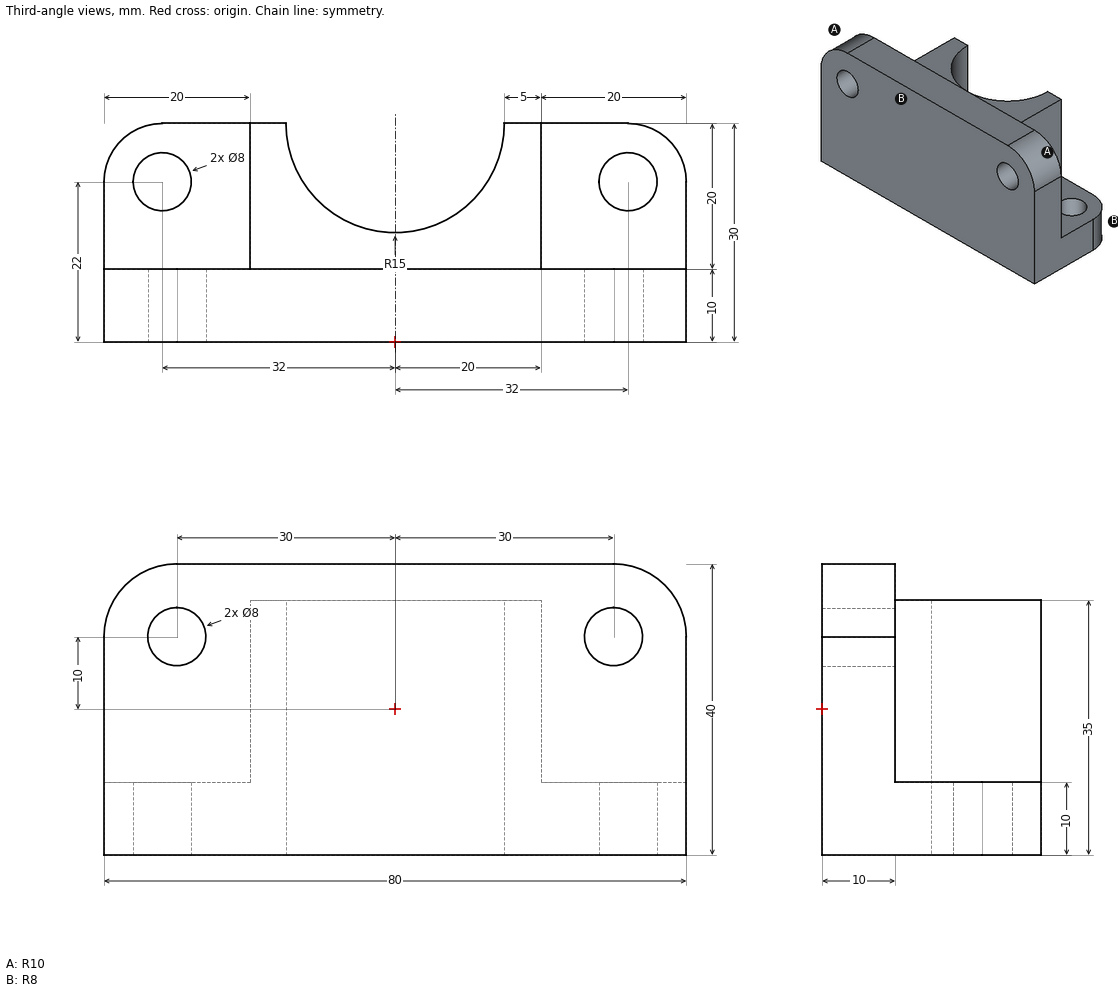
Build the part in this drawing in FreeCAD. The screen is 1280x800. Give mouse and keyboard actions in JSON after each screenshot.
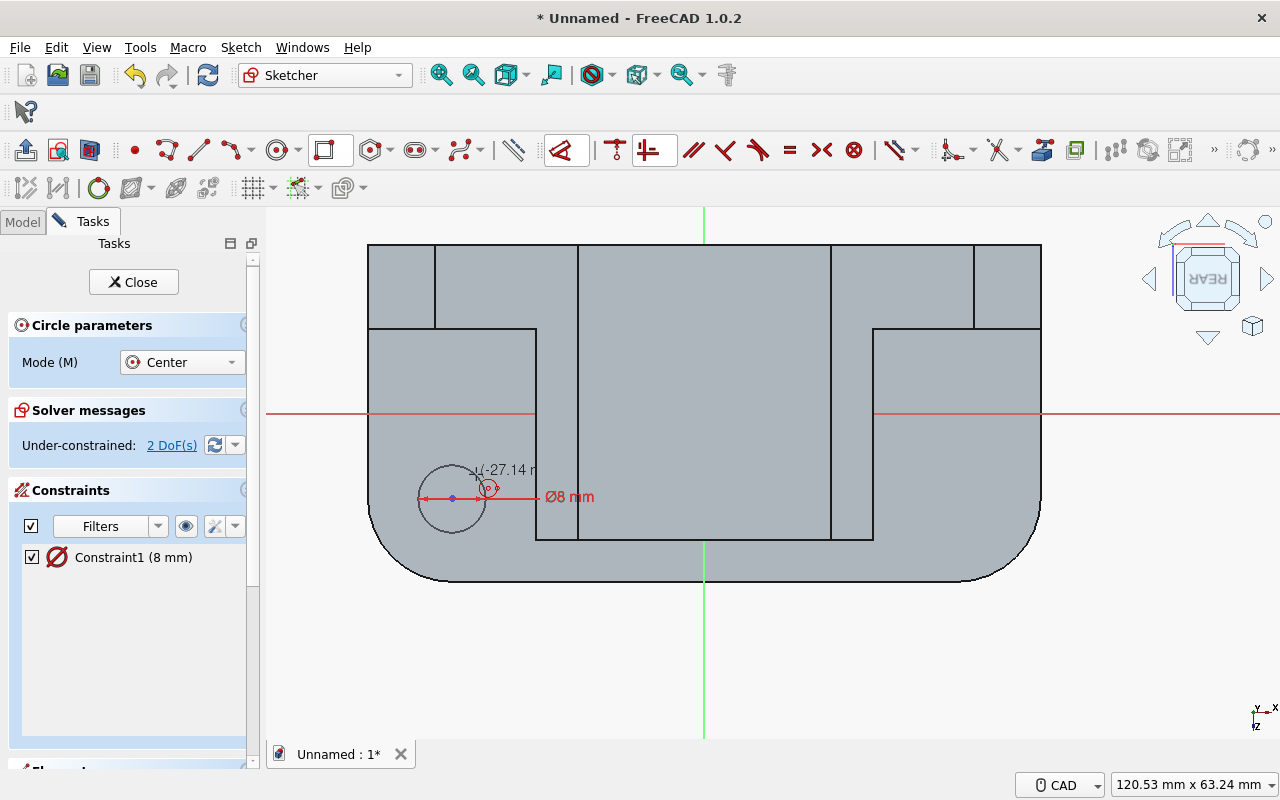
{"action": "left_click", "coordinate": [957, 498]}
{"action": "mouse_move", "coordinate": [980, 474]}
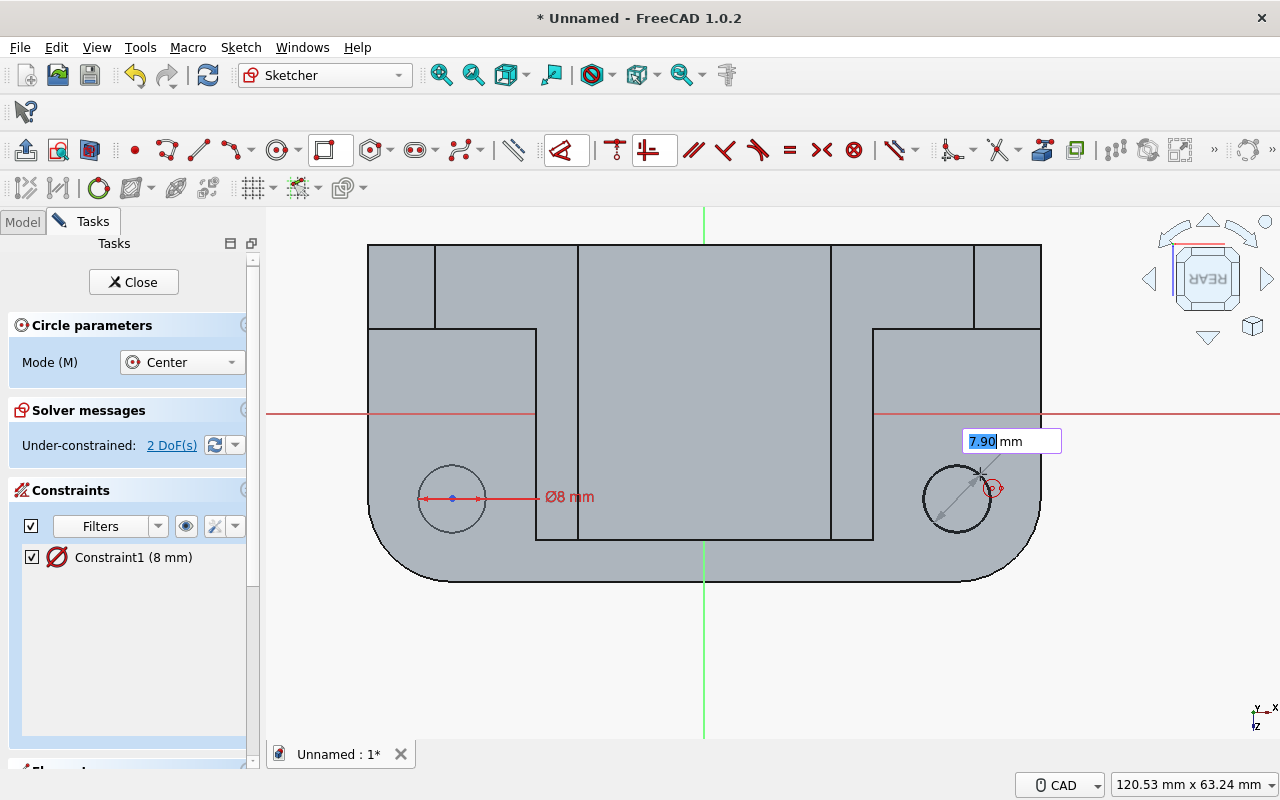
{"action": "type", "text": "8"}
{"action": "key", "text": "Return"}
{"action": "key", "text": "Escape"}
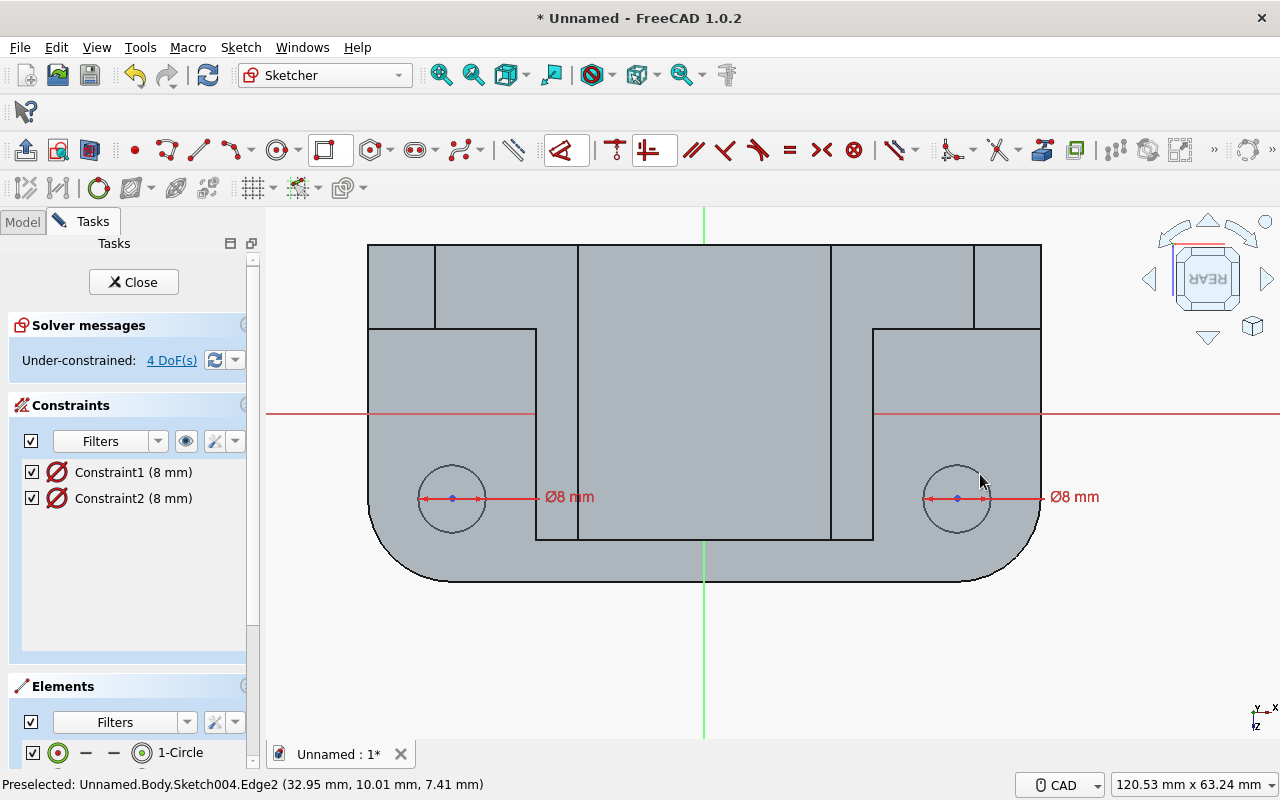
{"action": "left_click", "coordinate": [452, 499]}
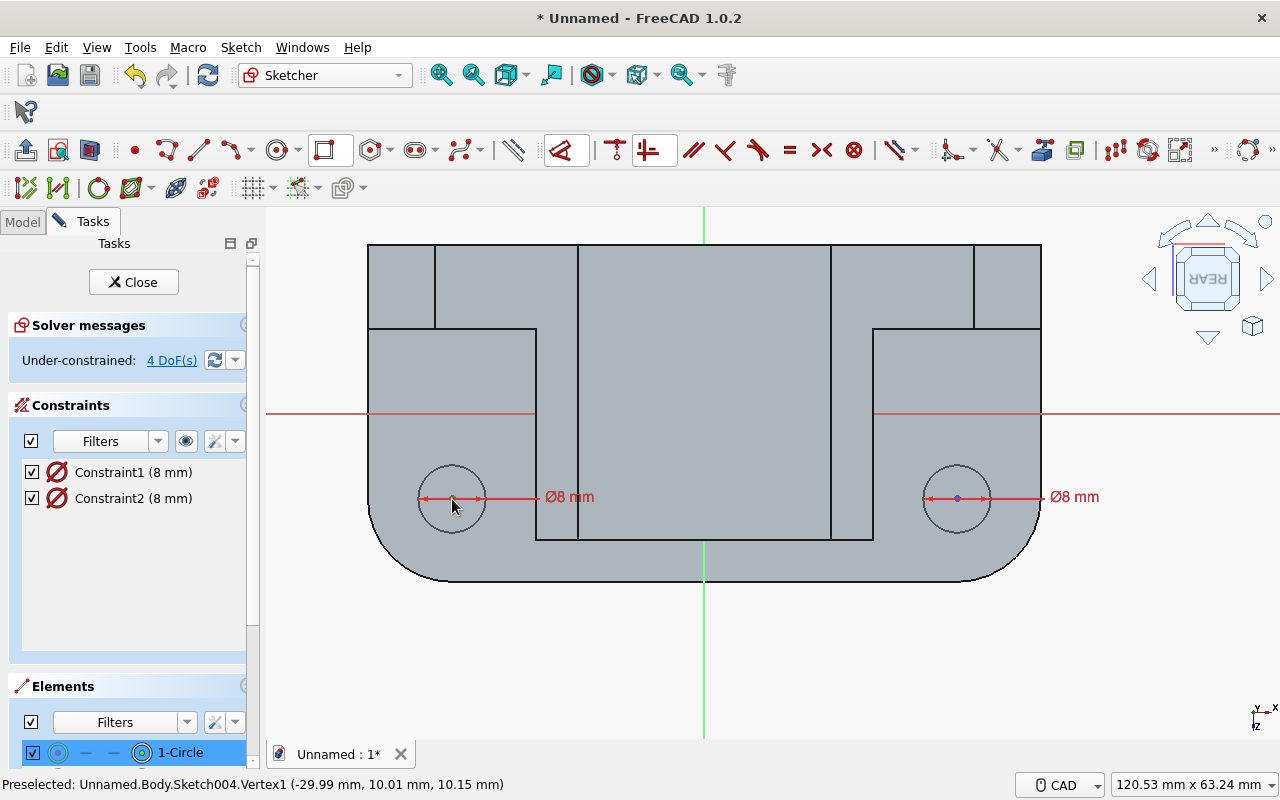
{"action": "left_click", "coordinate": [957, 499]}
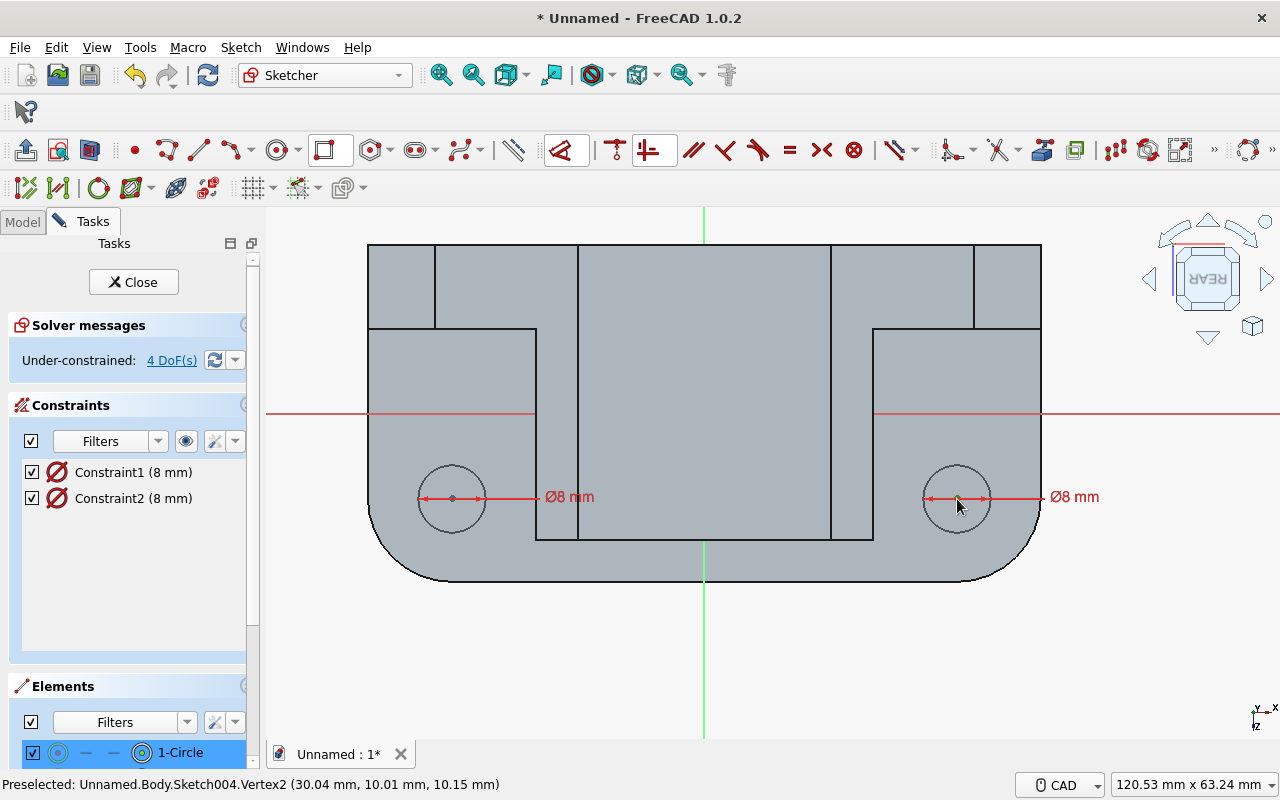
{"action": "key", "text": "h"}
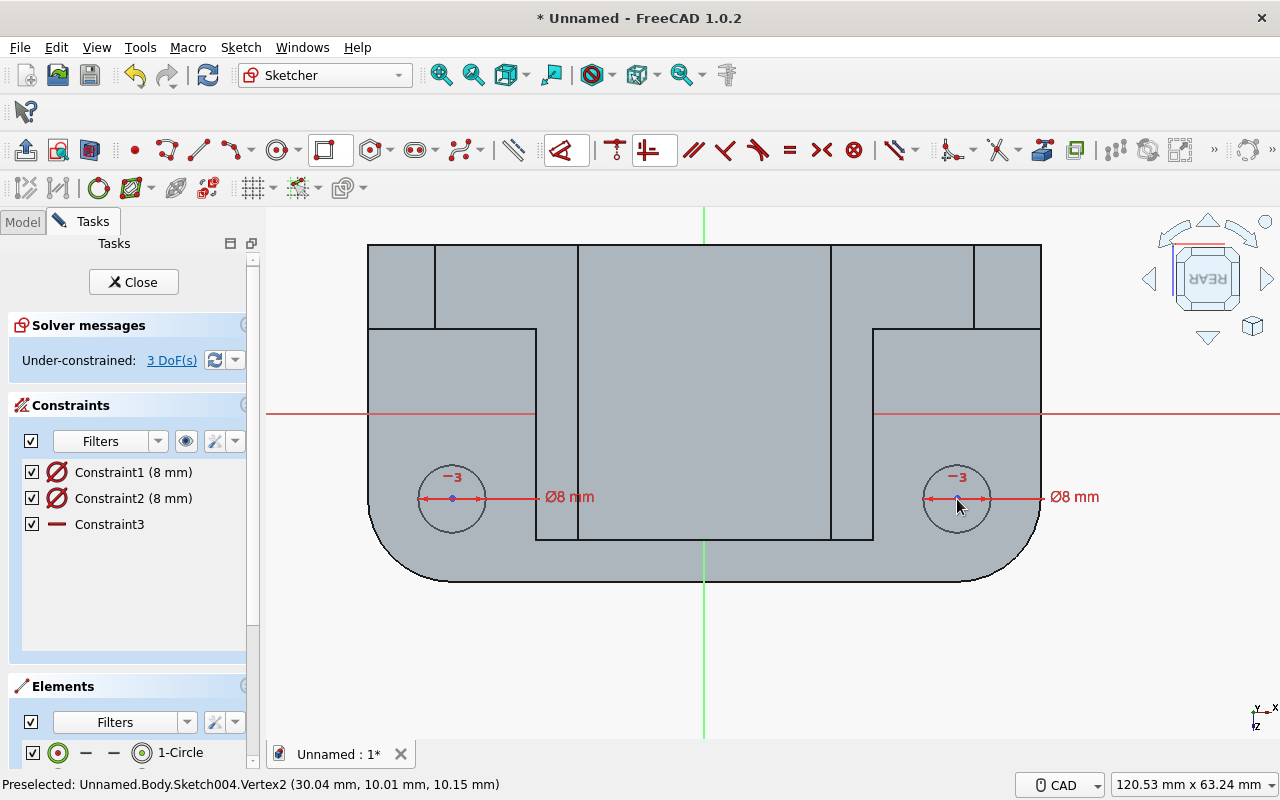
{"action": "left_click", "coordinate": [452, 499]}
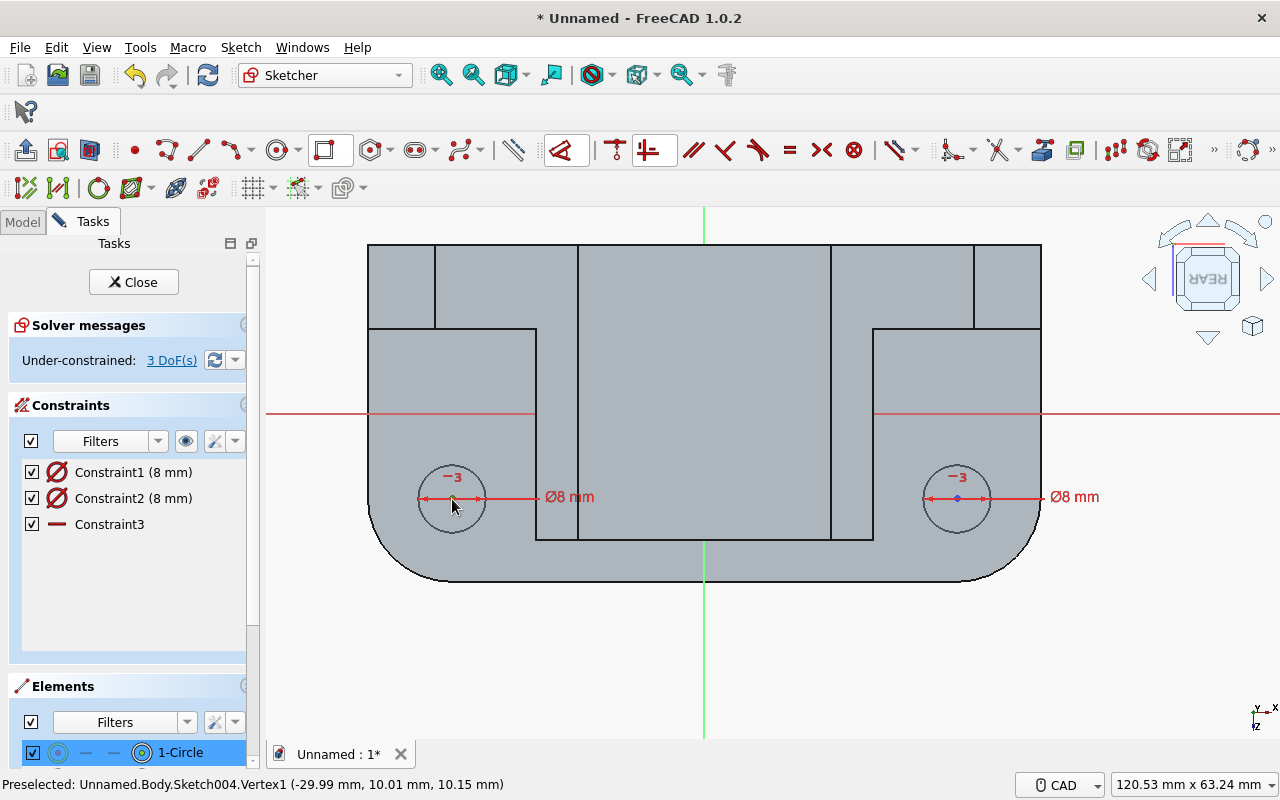
{"action": "left_click", "coordinate": [584, 150]}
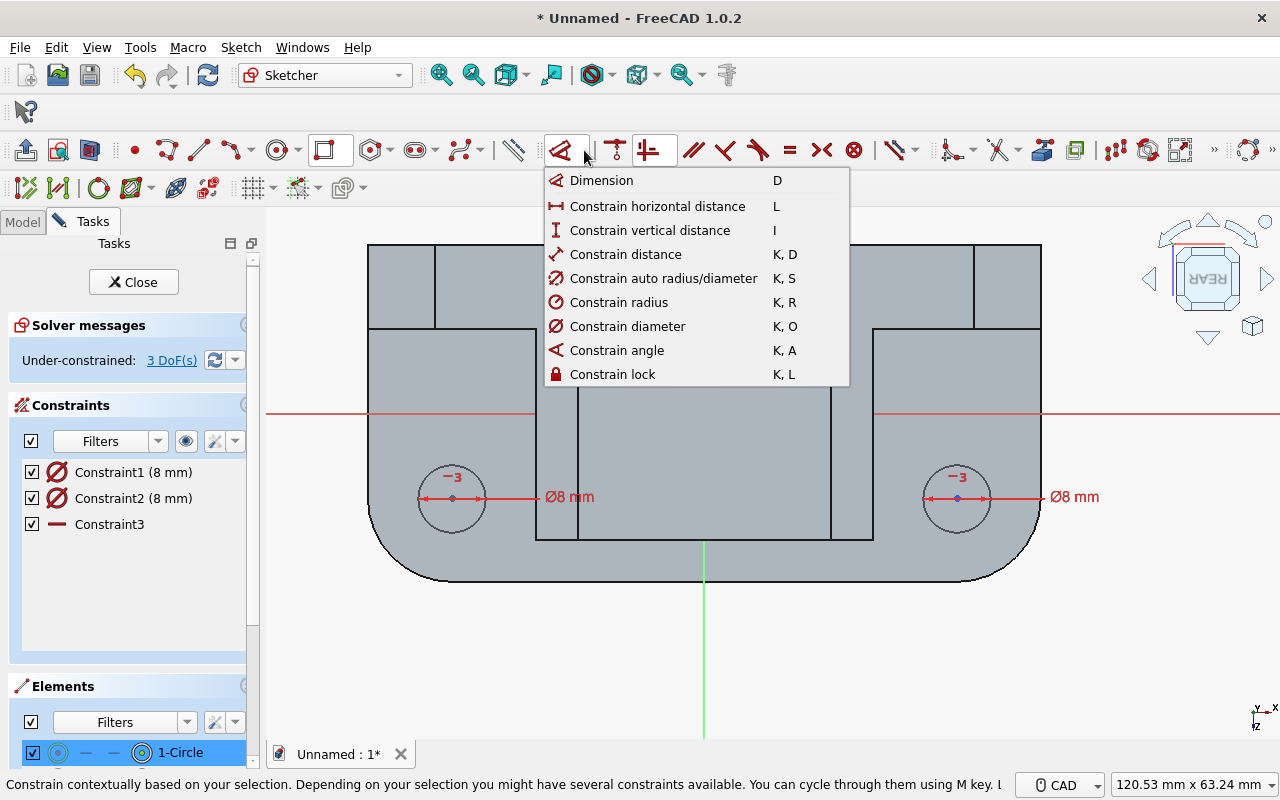
{"action": "left_click", "coordinate": [697, 206]}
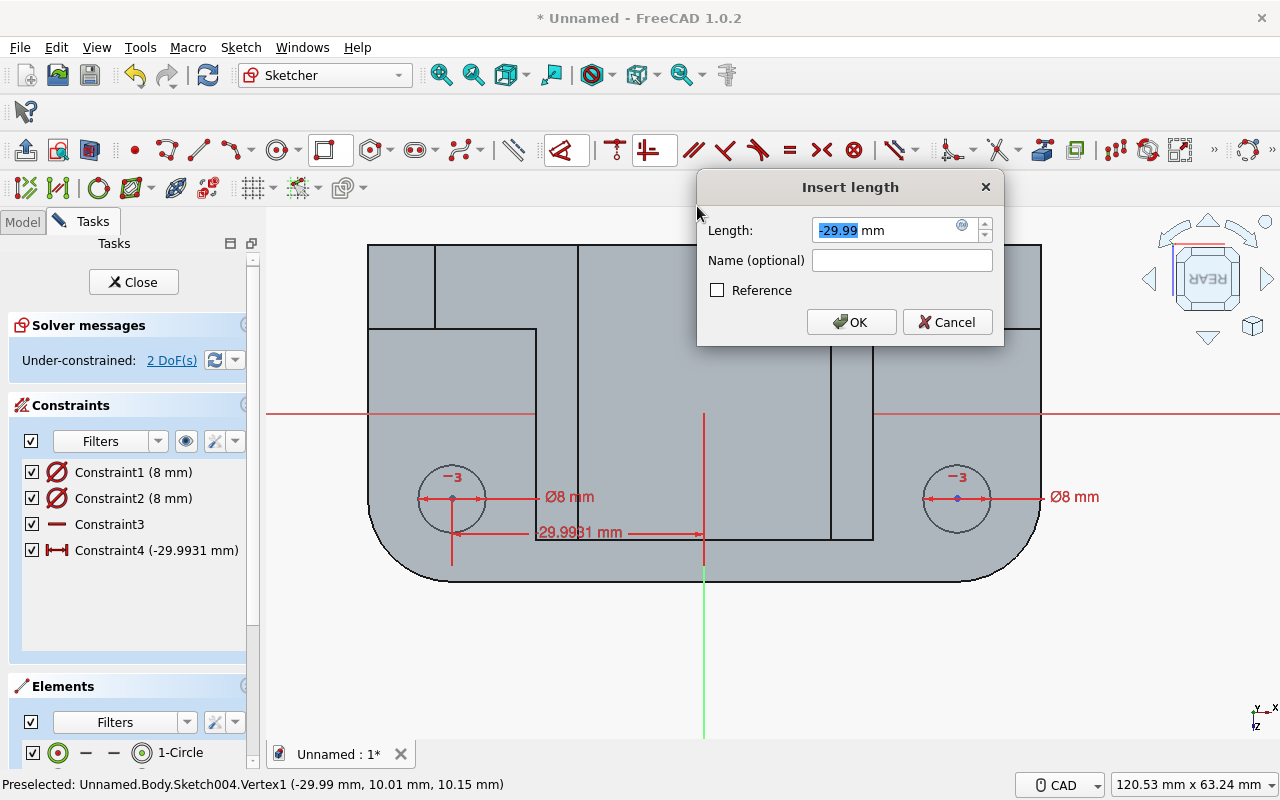
{"action": "type", "text": "-30"}
{"action": "key", "text": "Return"}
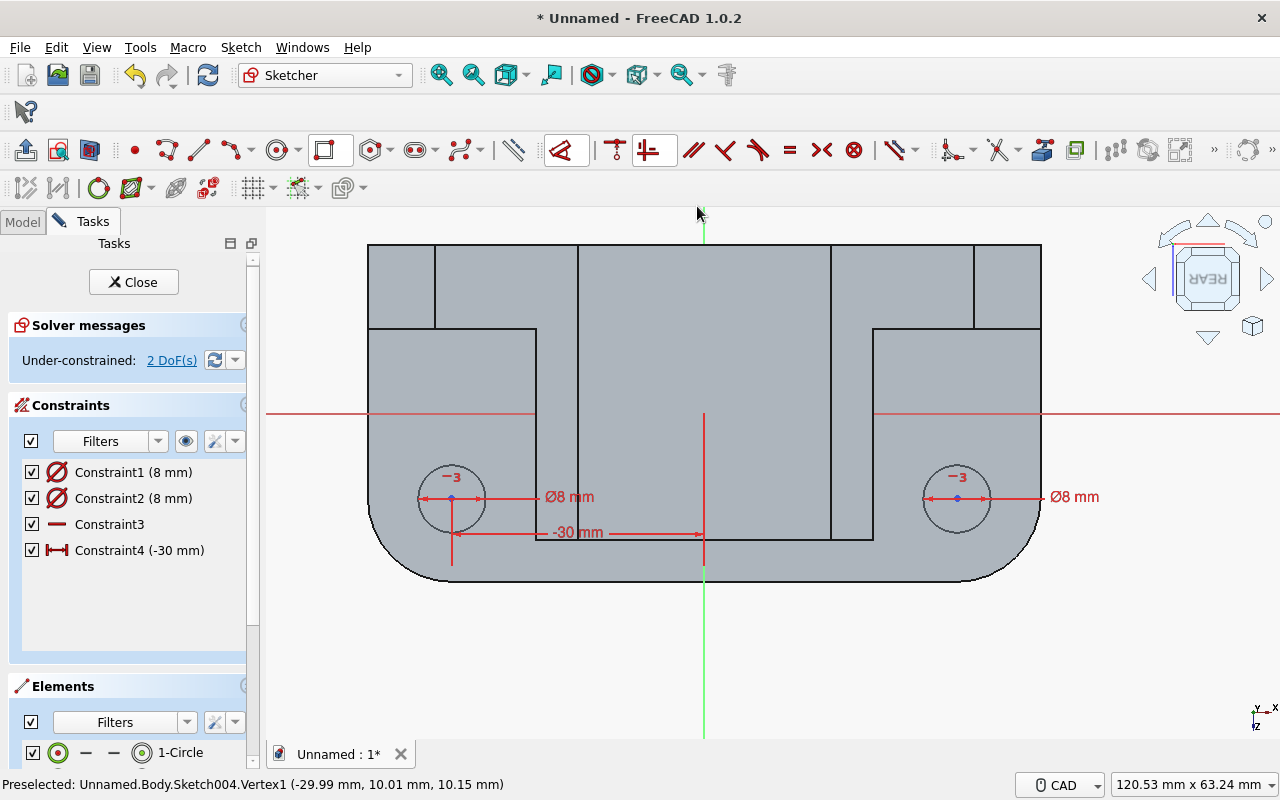
{"action": "left_click", "coordinate": [452, 499]}